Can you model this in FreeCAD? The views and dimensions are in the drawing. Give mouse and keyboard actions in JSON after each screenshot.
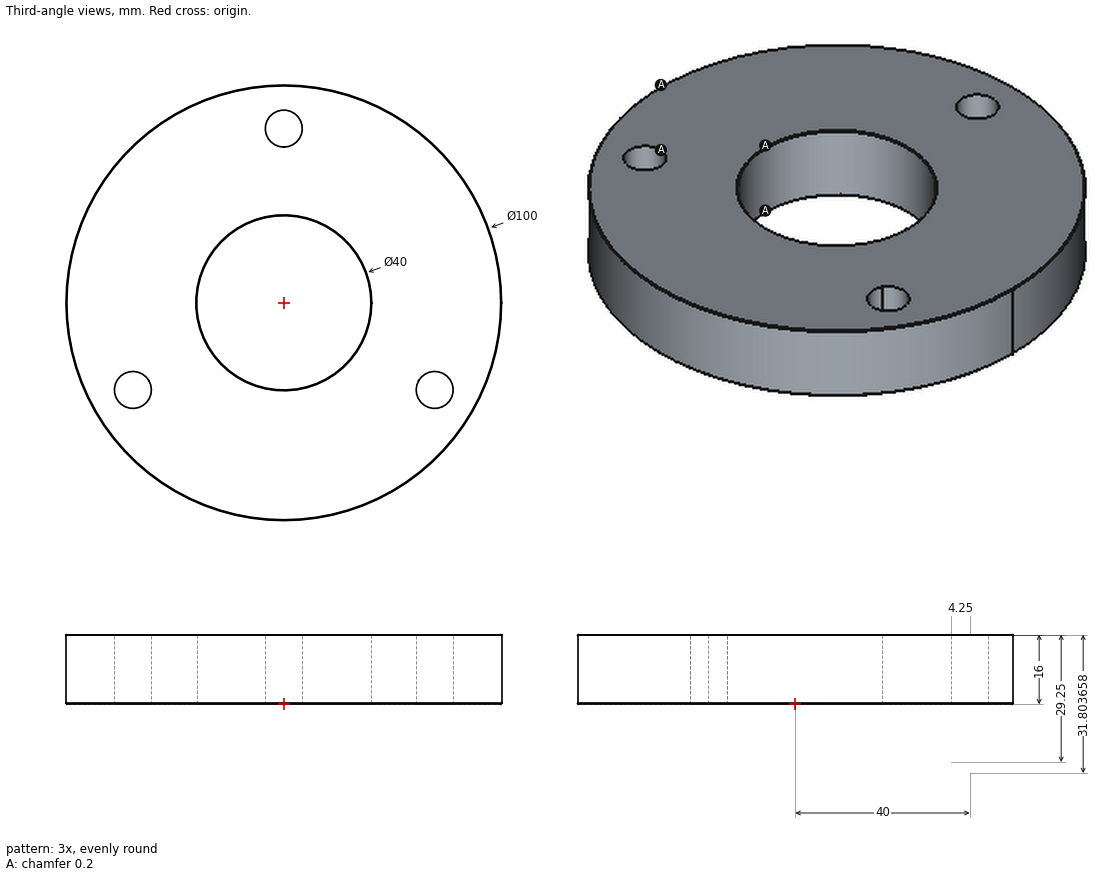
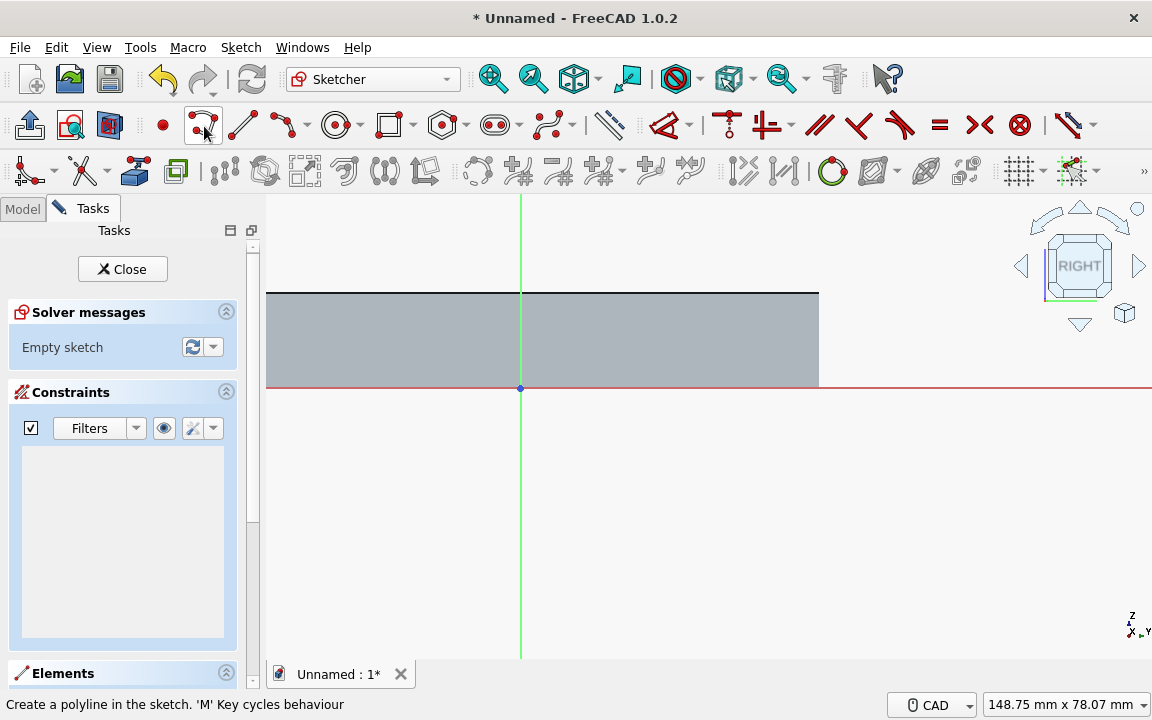
{"action": "left_click", "coordinate": [734, 467]}
{"action": "left_click", "coordinate": [759, 483]}
{"action": "left_click", "coordinate": [759, 293]}
{"action": "left_click", "coordinate": [734, 293]}
{"action": "left_click", "coordinate": [734, 468]}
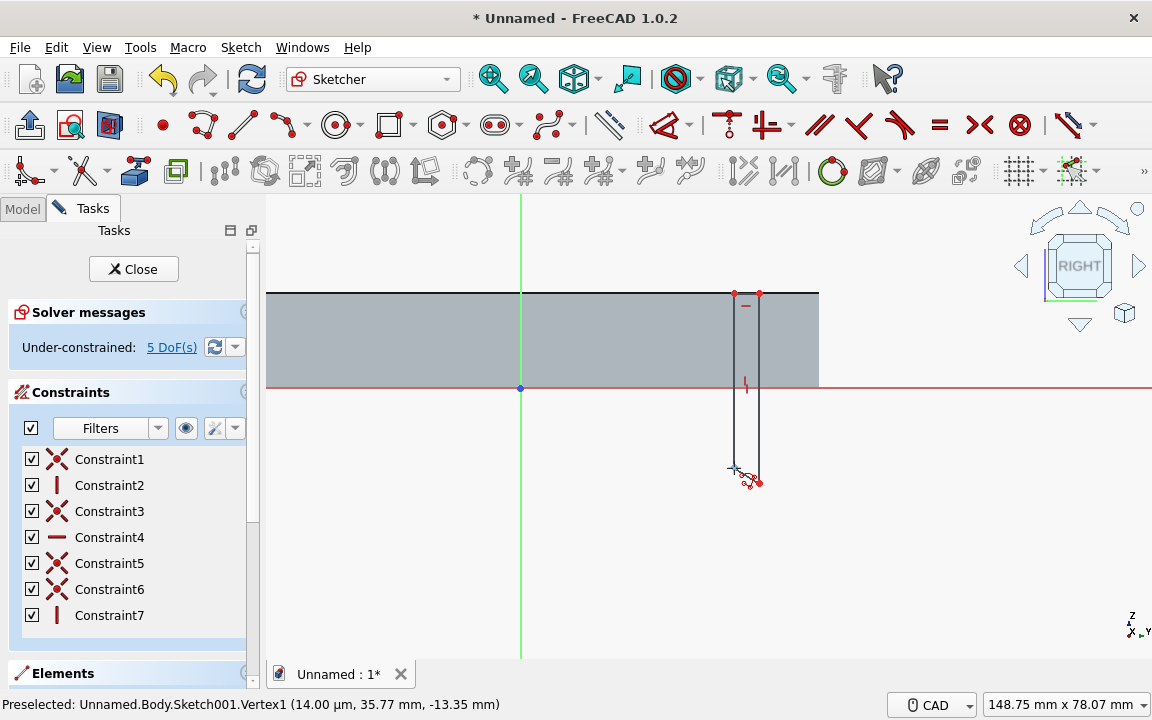
{"action": "left_click", "coordinate": [244, 126]}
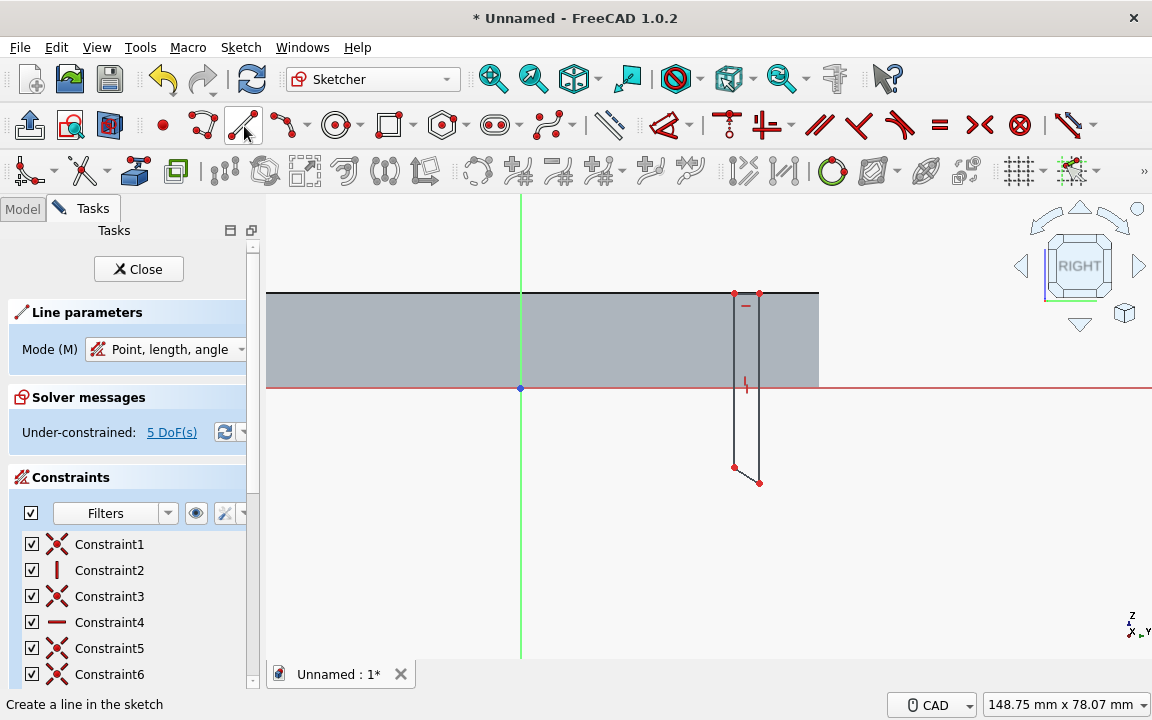
{"action": "left_click", "coordinate": [759, 502]}
{"action": "left_click", "coordinate": [759, 558]}
{"action": "key", "text": "Escape"}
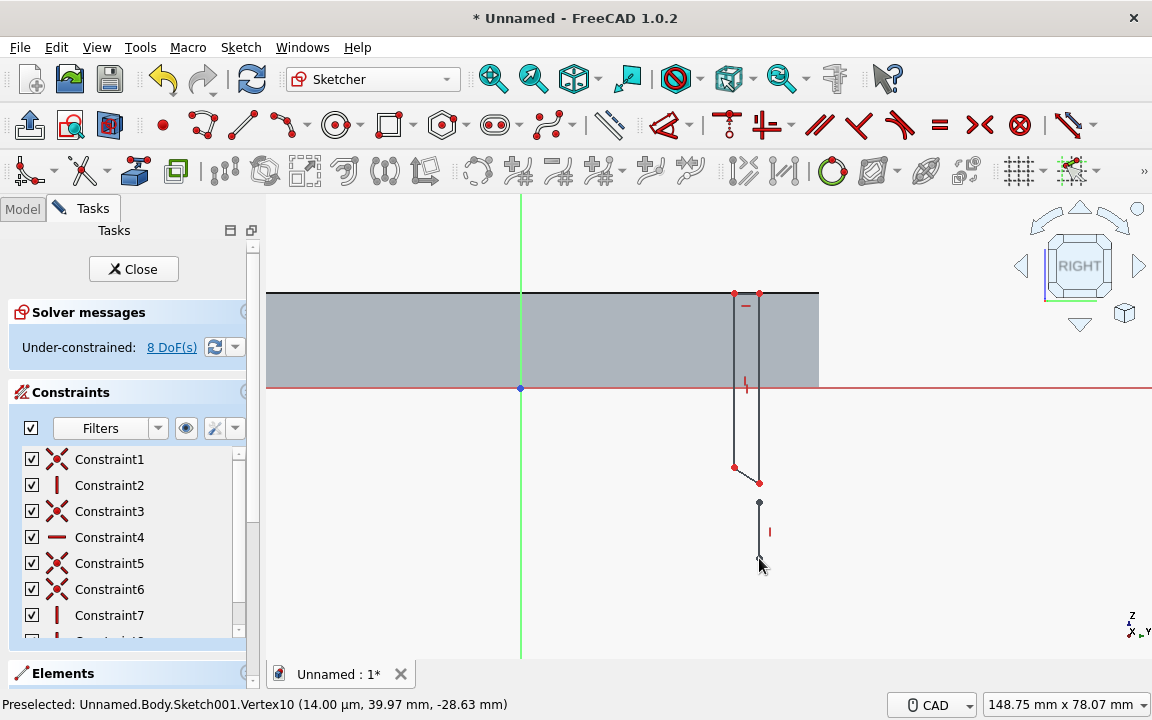
{"action": "left_click", "coordinate": [759, 520]}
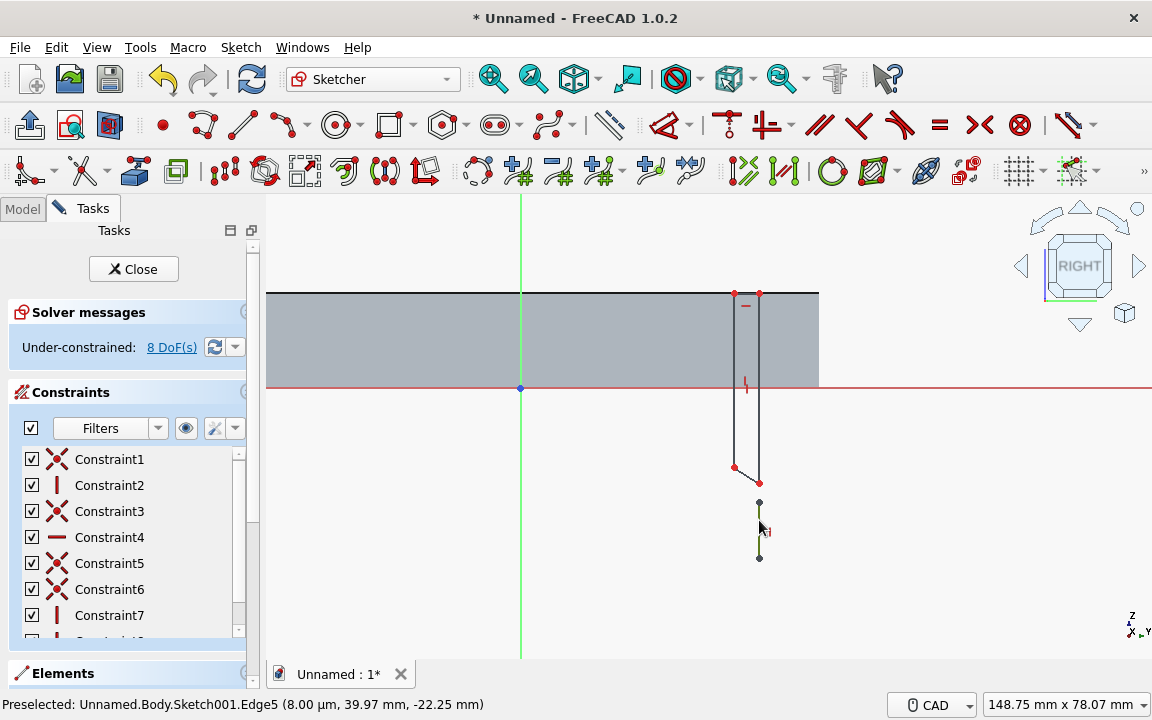
{"action": "left_click", "coordinate": [610, 126]}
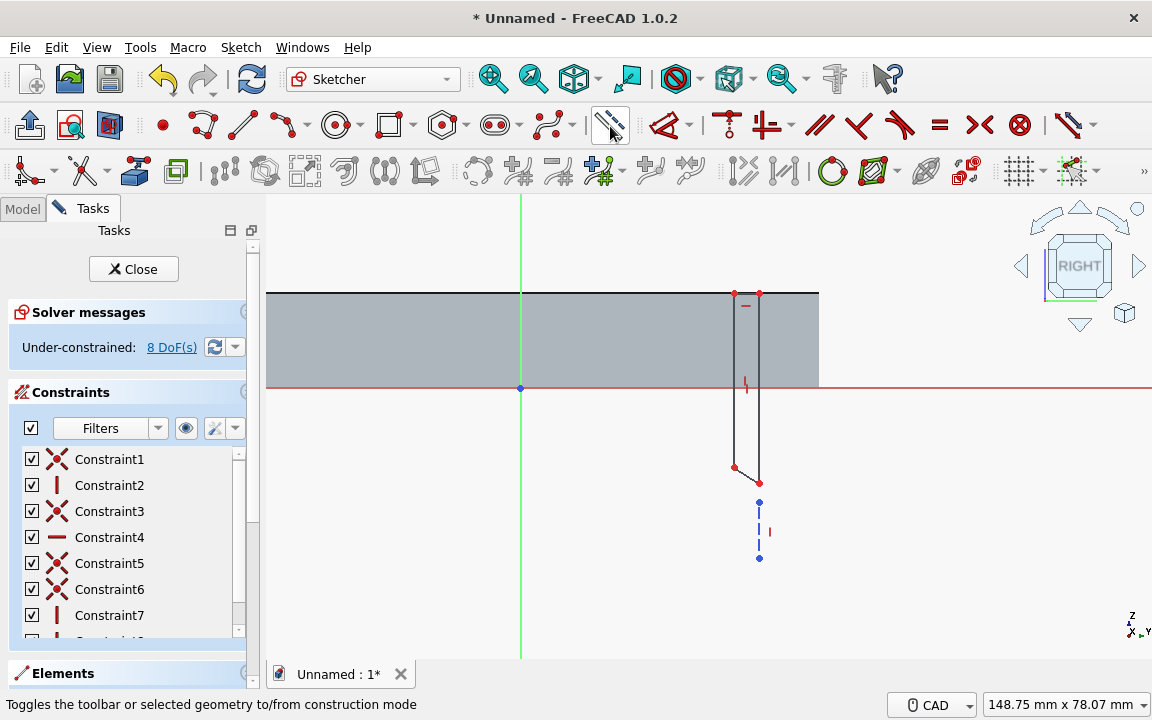
{"action": "left_click", "coordinate": [664, 126]}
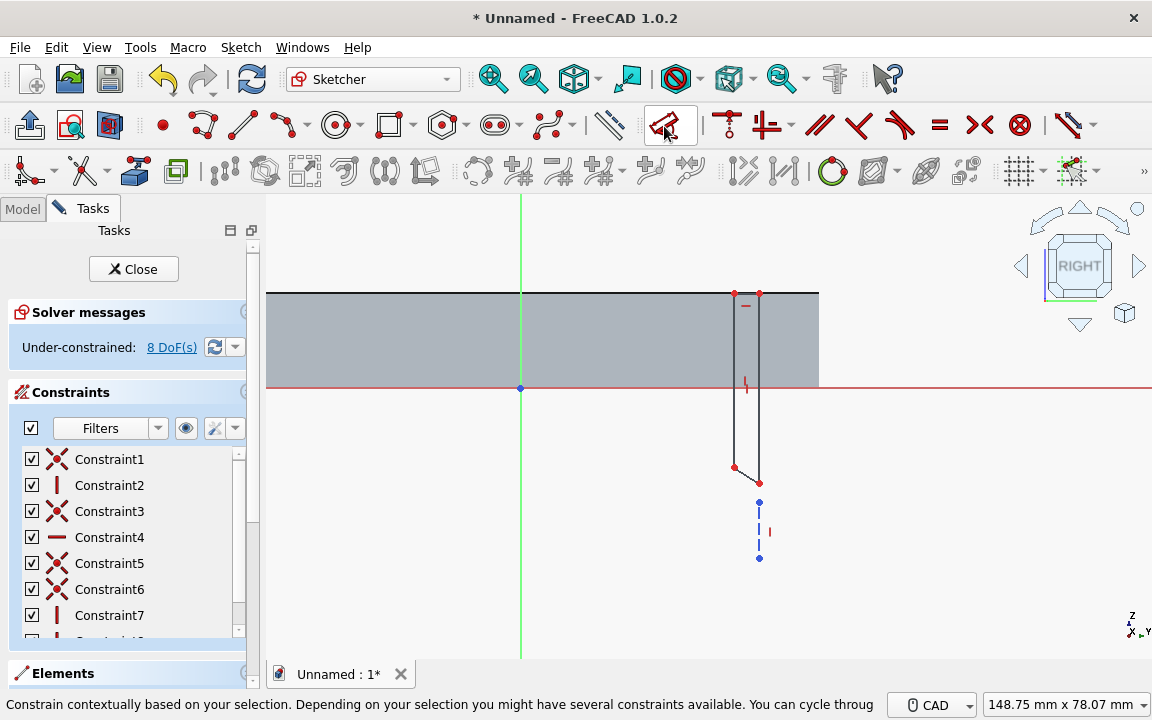
{"action": "left_click", "coordinate": [759, 484]}
{"action": "left_click", "coordinate": [640, 518]}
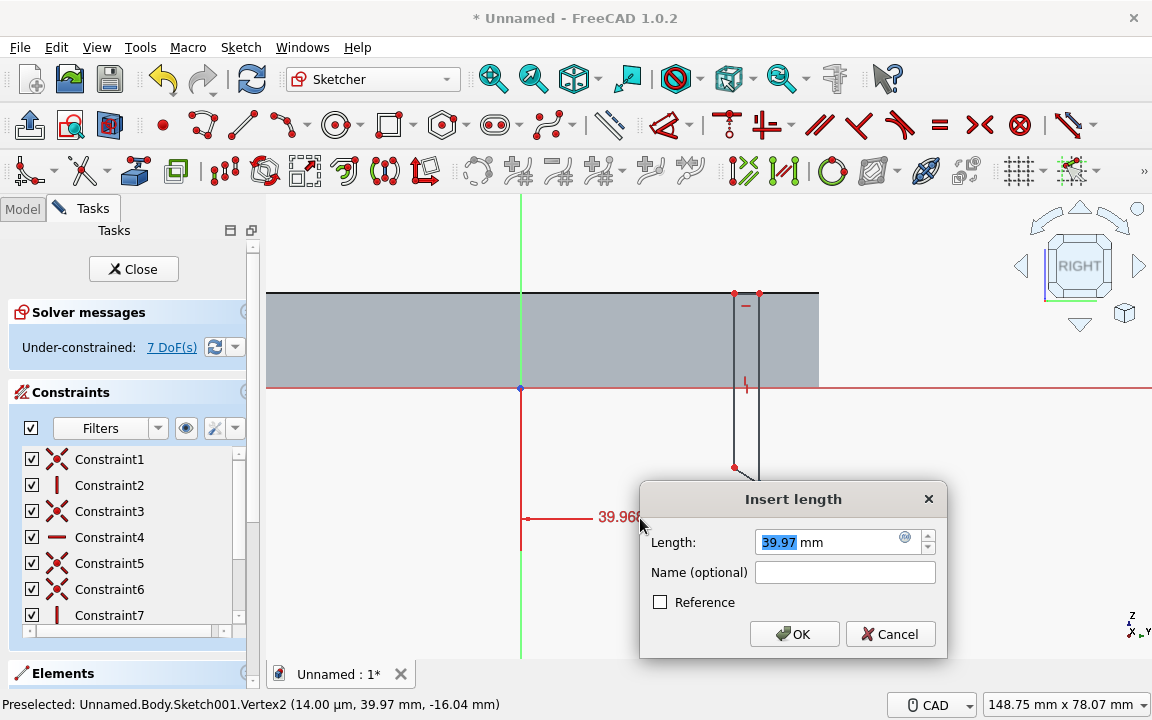
{"action": "type", "text": "40"}
{"action": "key", "text": "Return"}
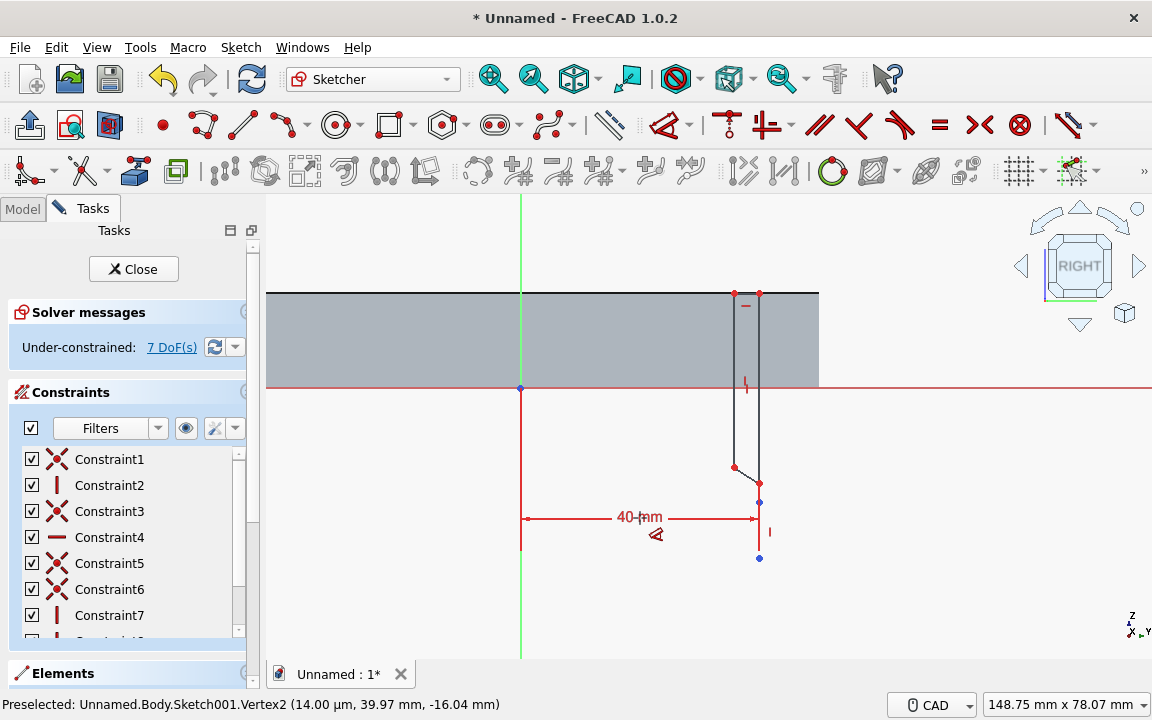
{"action": "left_click", "coordinate": [759, 294]}
{"action": "left_click", "coordinate": [793, 341]}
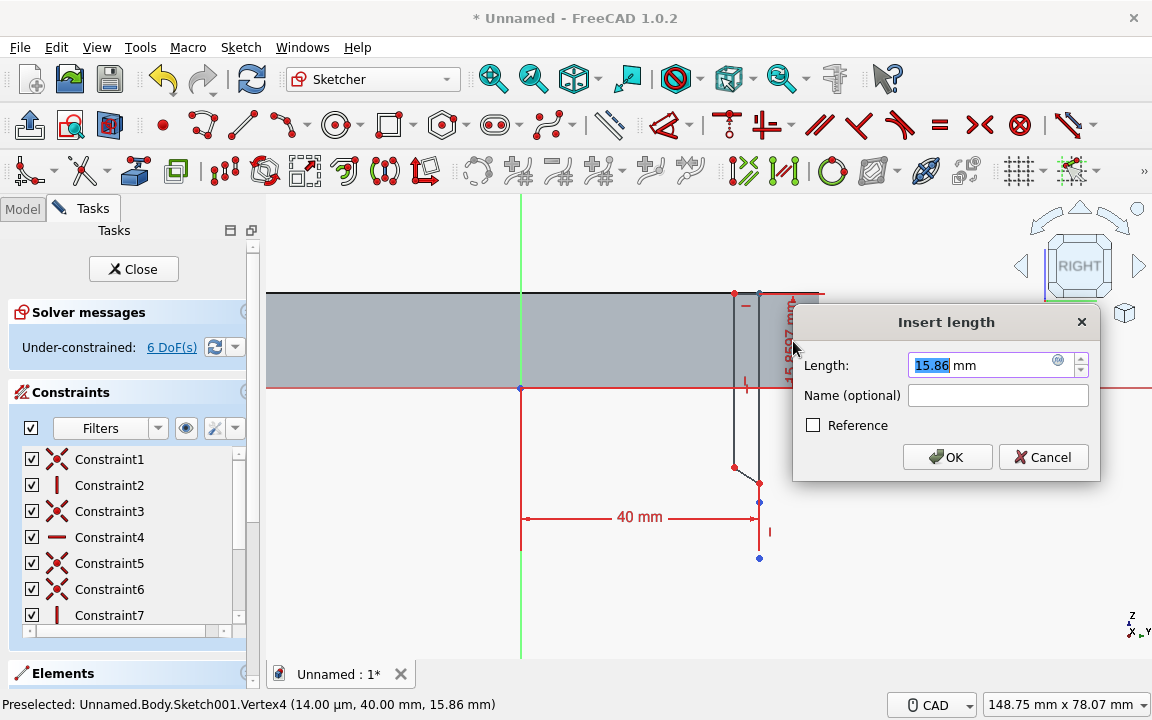
{"action": "type", "text": "16"}
{"action": "key", "text": "Return"}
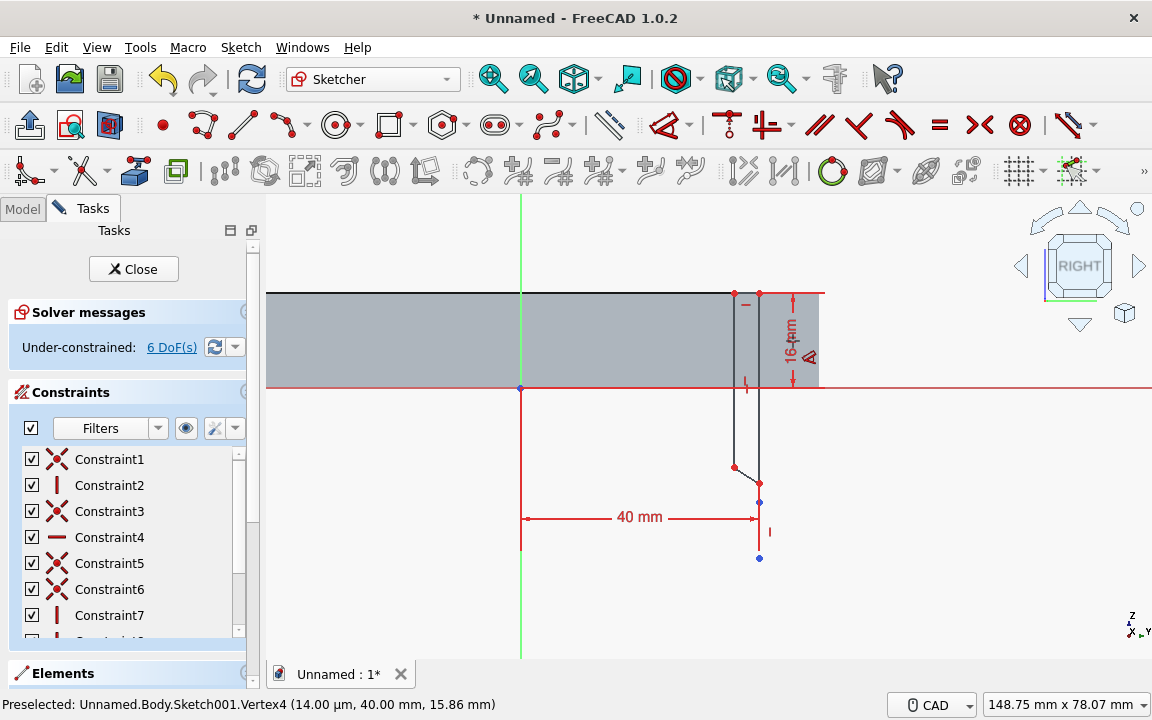
{"action": "left_click", "coordinate": [759, 503]}
{"action": "left_click", "coordinate": [557, 537]}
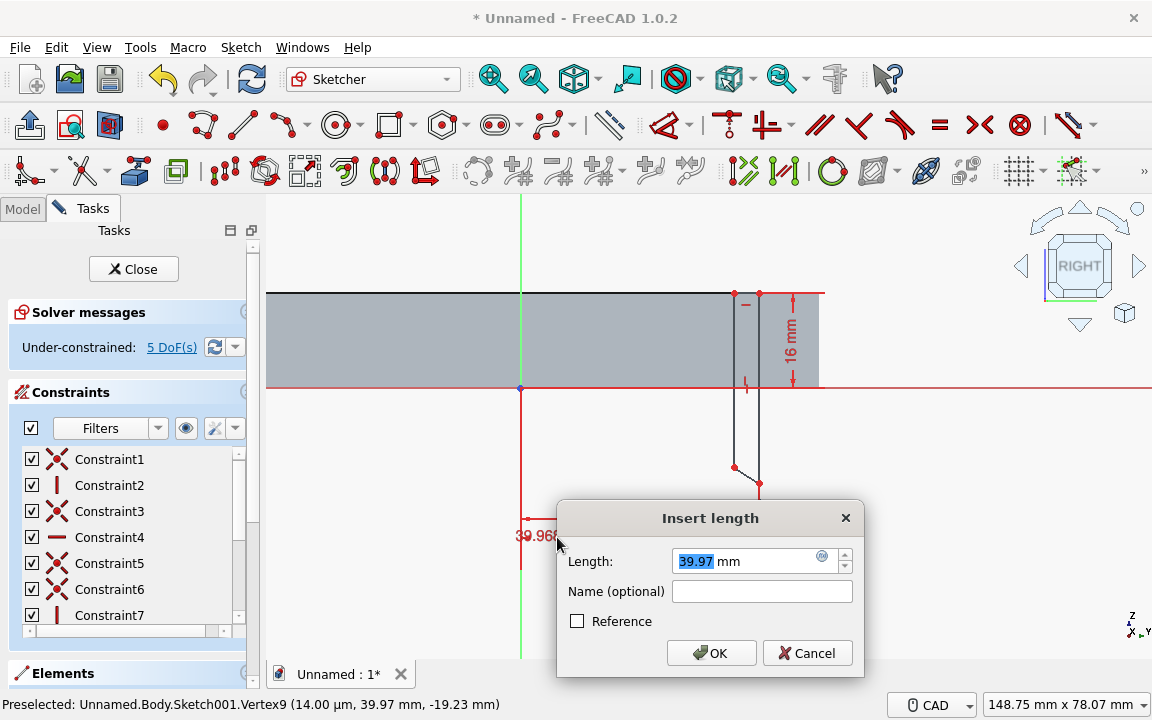
{"action": "type", "text": "40"}
{"action": "key", "text": "Return"}